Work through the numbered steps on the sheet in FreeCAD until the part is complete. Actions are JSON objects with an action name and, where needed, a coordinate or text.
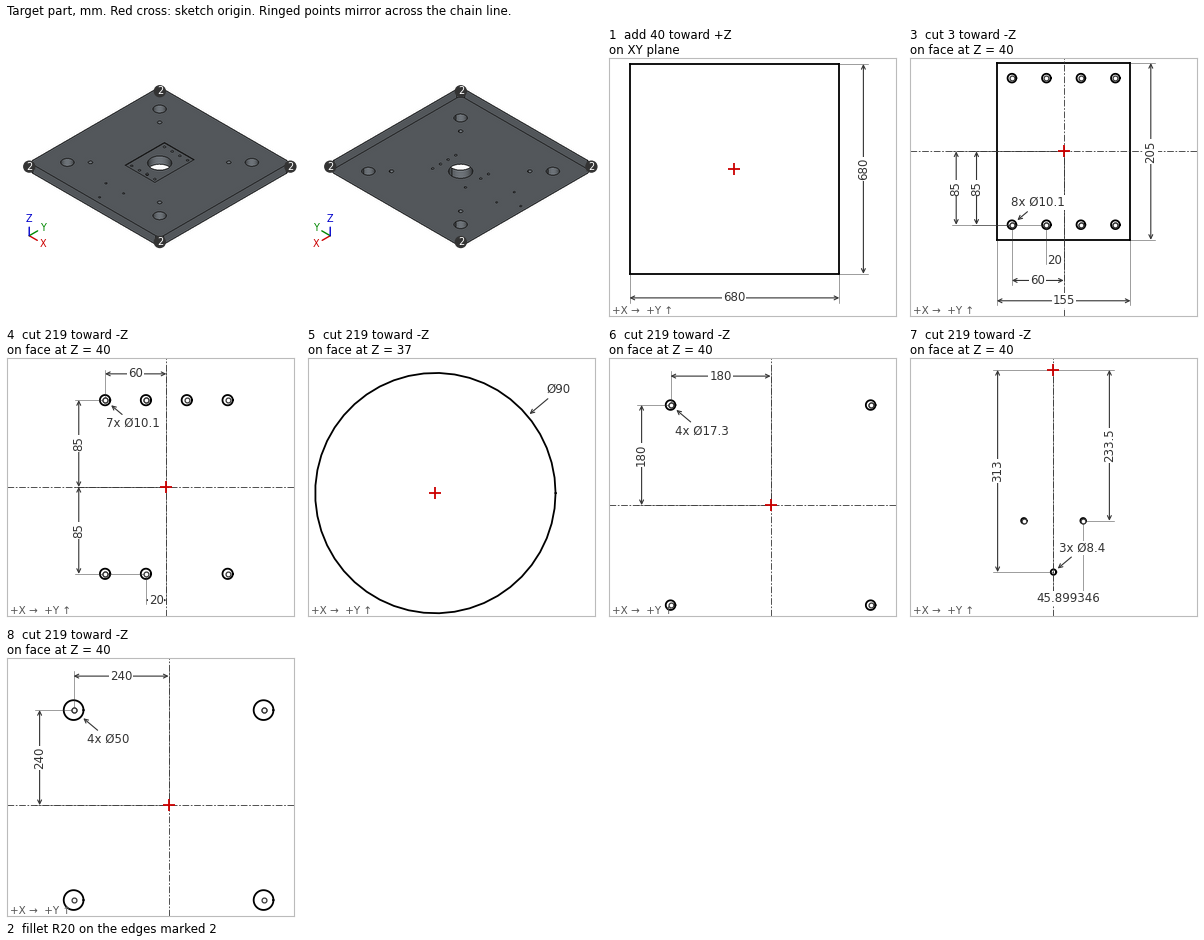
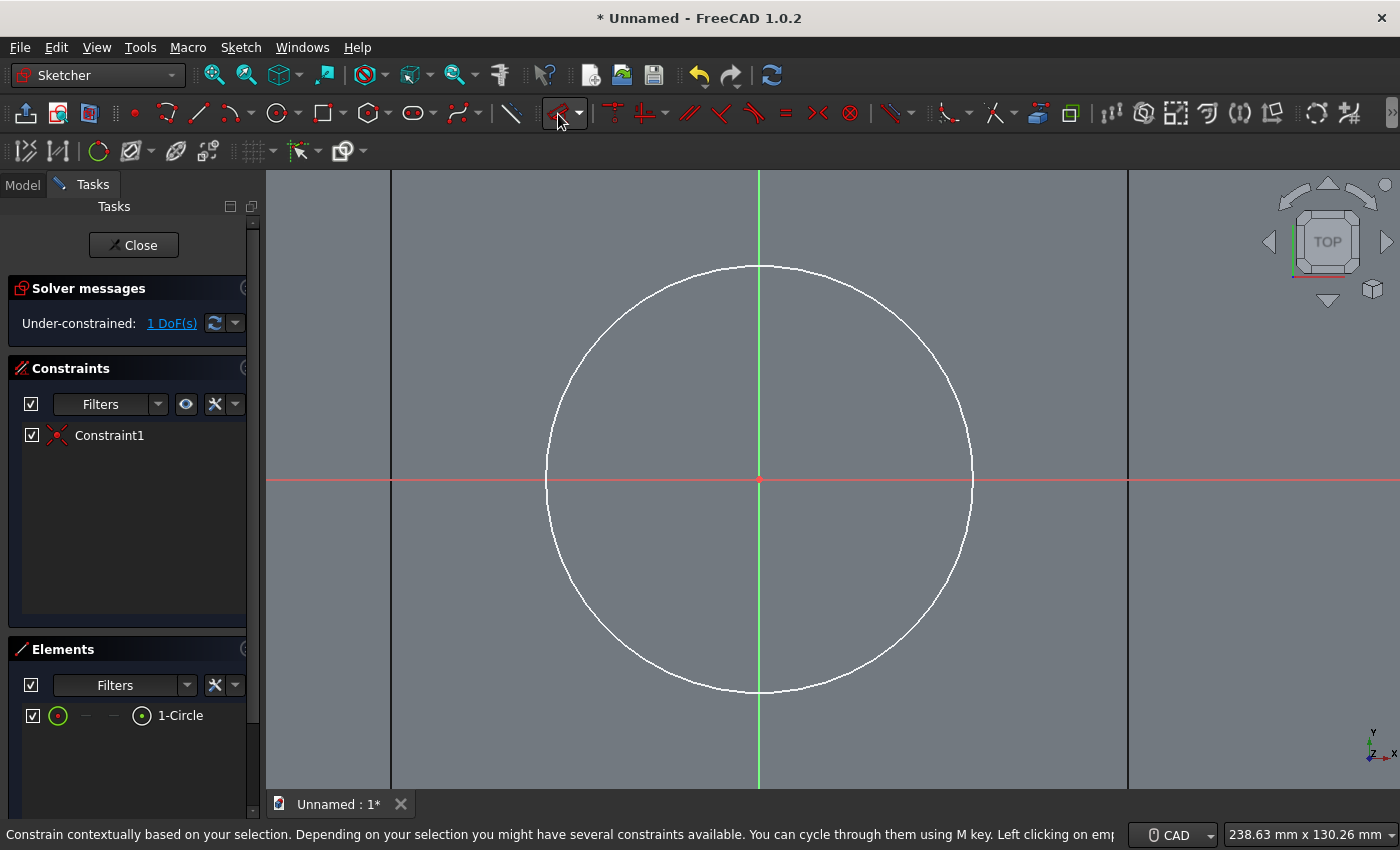
{"action": "left_click", "coordinate": [910, 328]}
{"action": "left_click", "coordinate": [933, 305]}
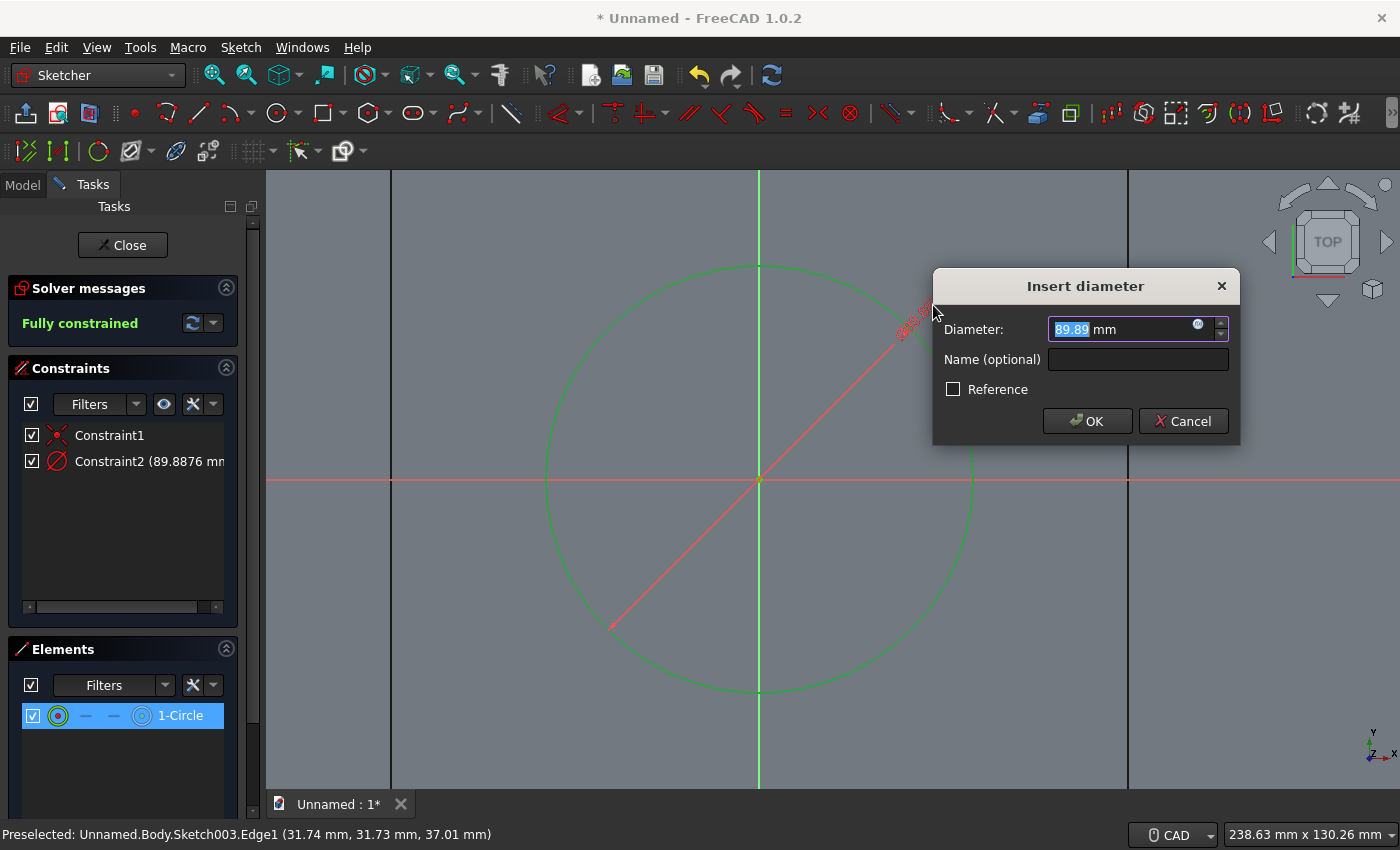
{"action": "type", "text": "90"}
{"action": "key", "text": "Return"}
{"action": "key", "text": "Escape"}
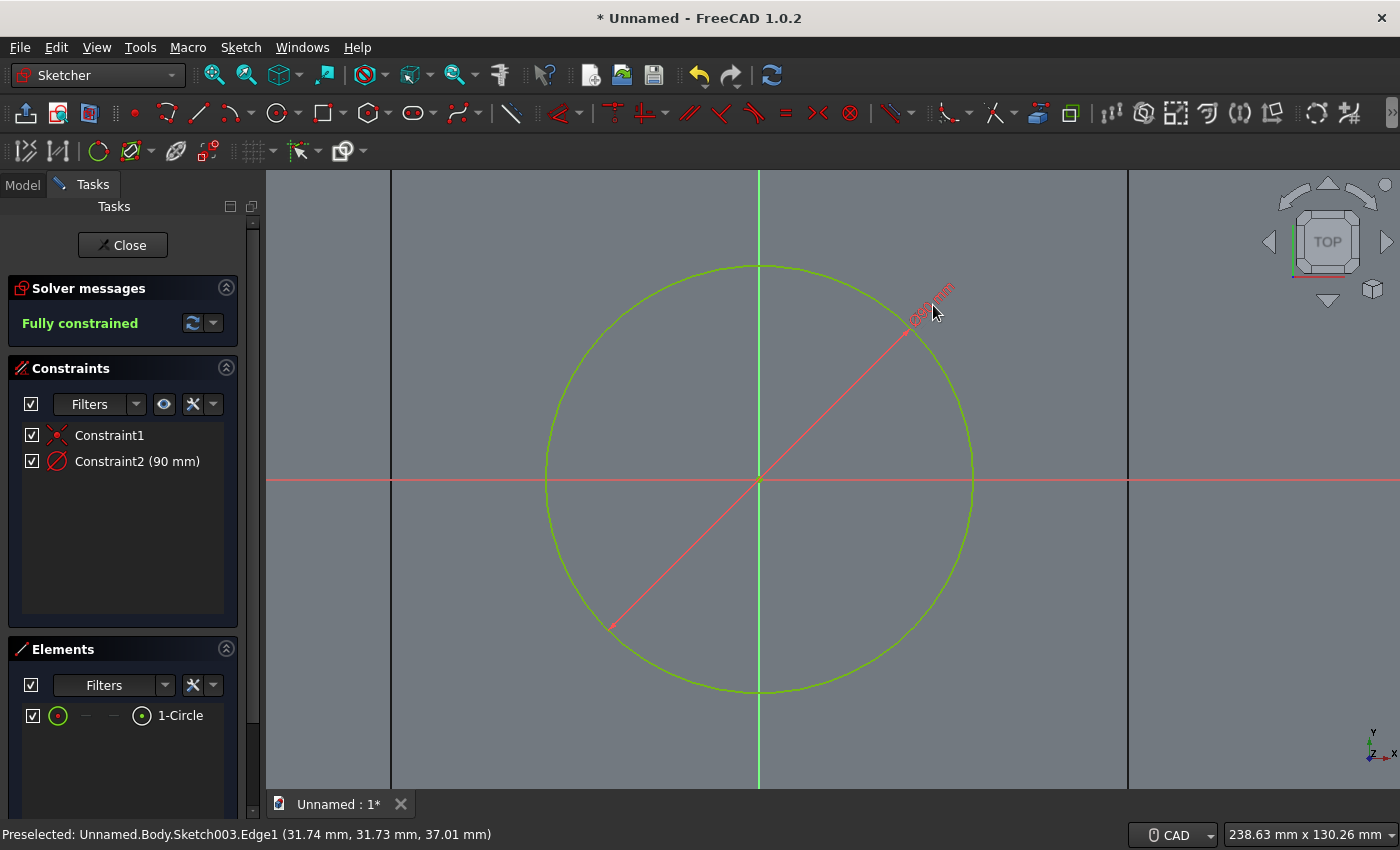
{"action": "left_click", "coordinate": [123, 245]}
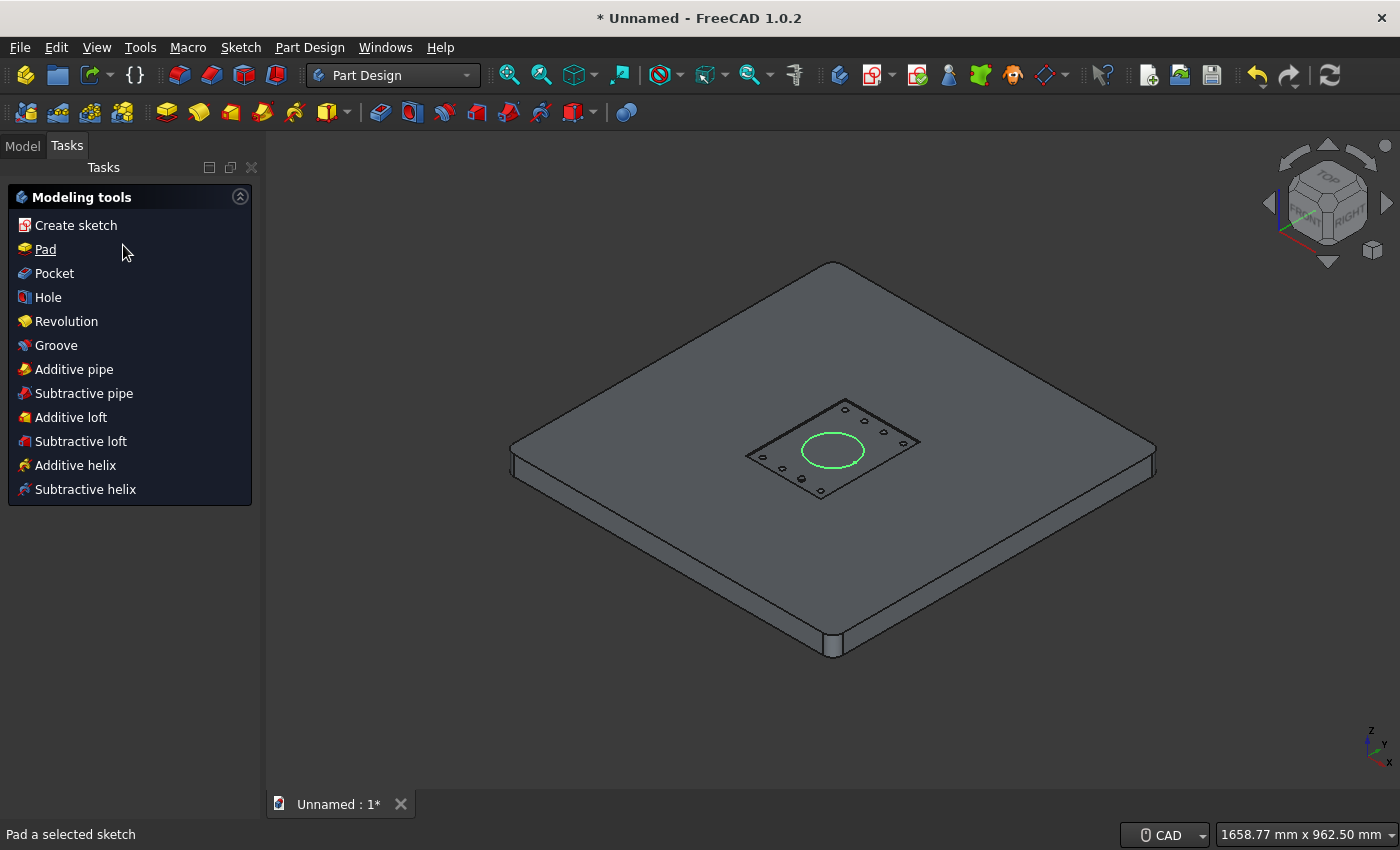
{"action": "left_click", "coordinate": [382, 112]}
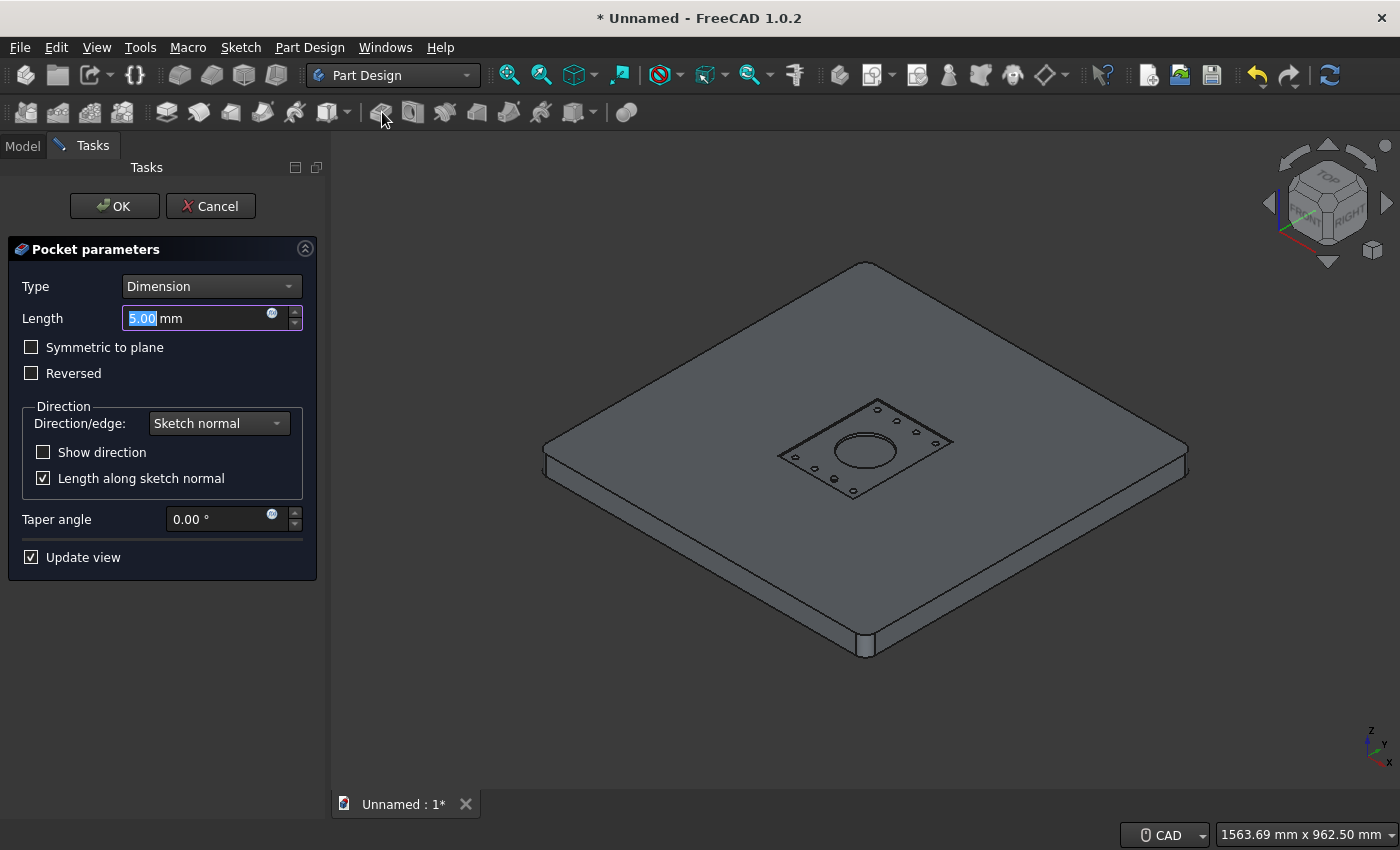
{"action": "type", "text": "219"}
{"action": "key", "text": "Tab"}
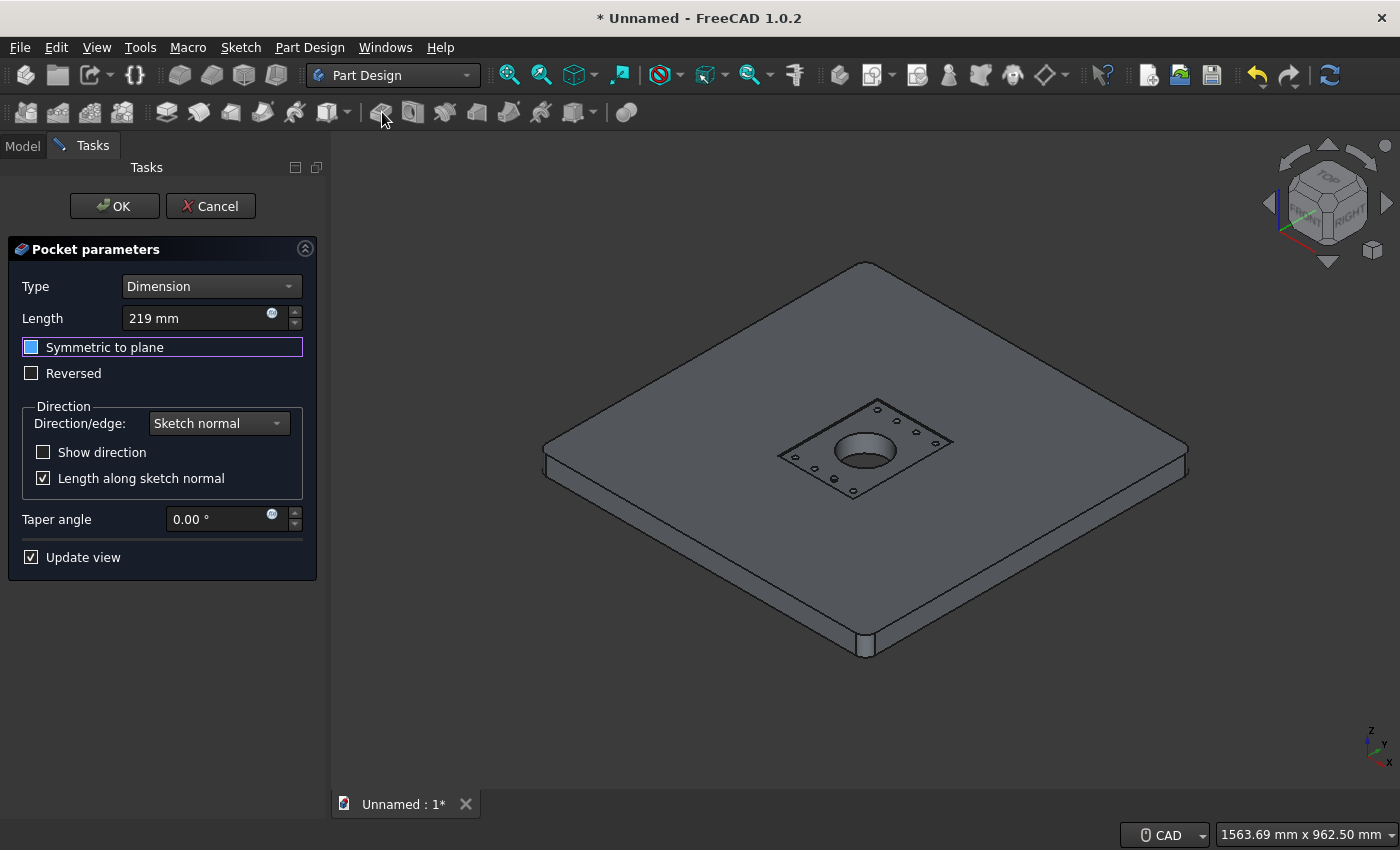
{"action": "left_click", "coordinate": [115, 206]}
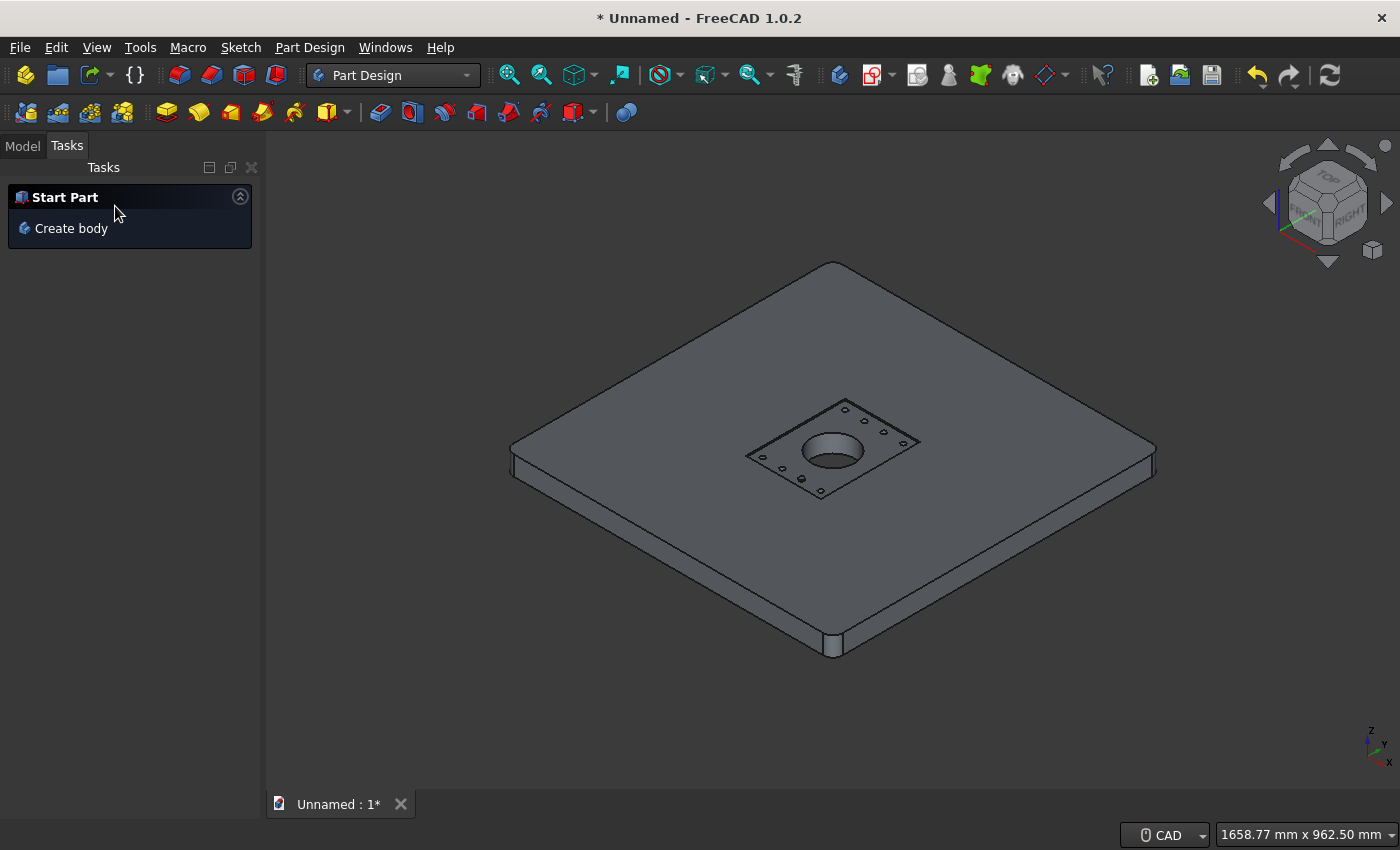
{"action": "left_click", "coordinate": [645, 448]}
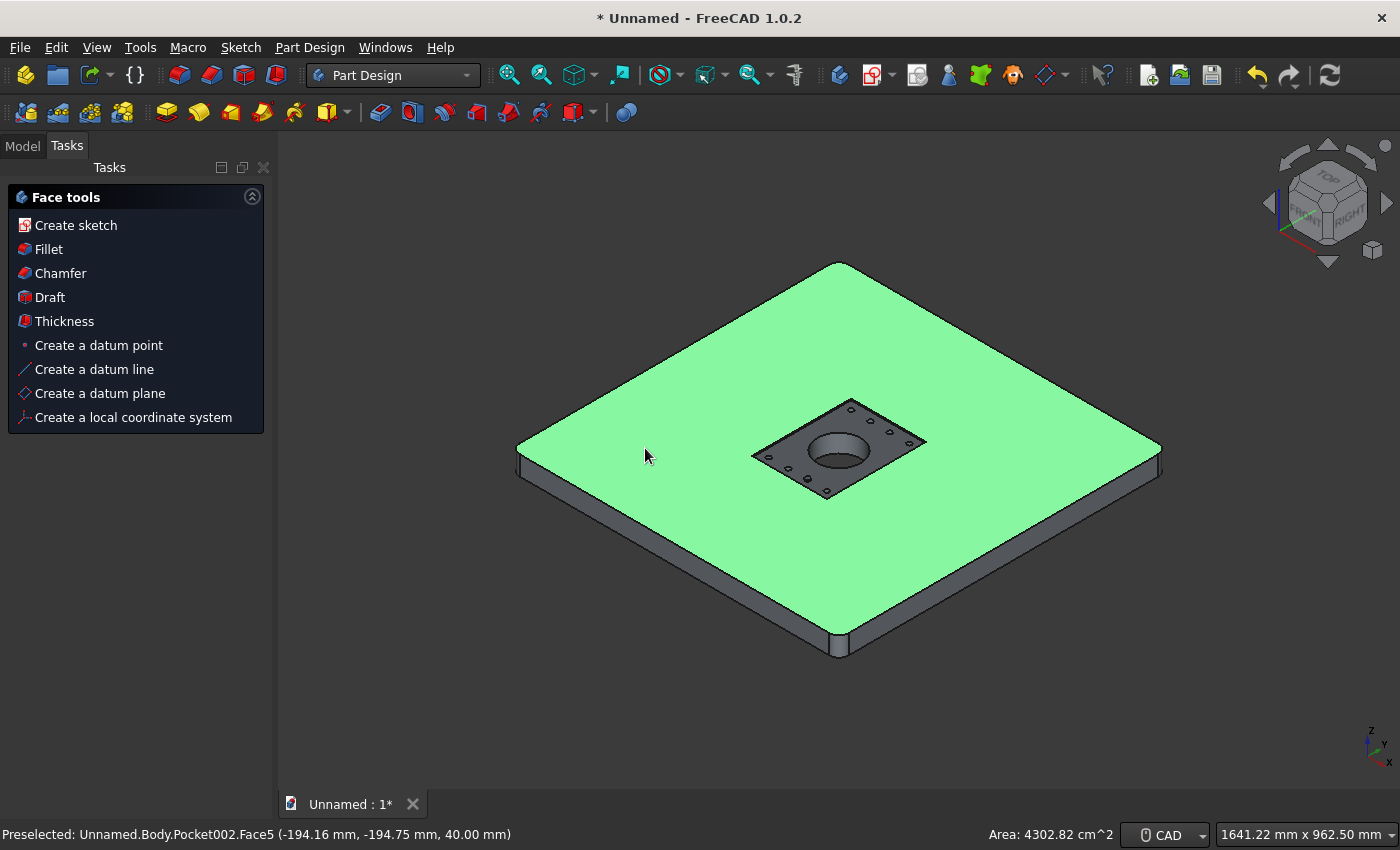
{"action": "left_click", "coordinate": [872, 76]}